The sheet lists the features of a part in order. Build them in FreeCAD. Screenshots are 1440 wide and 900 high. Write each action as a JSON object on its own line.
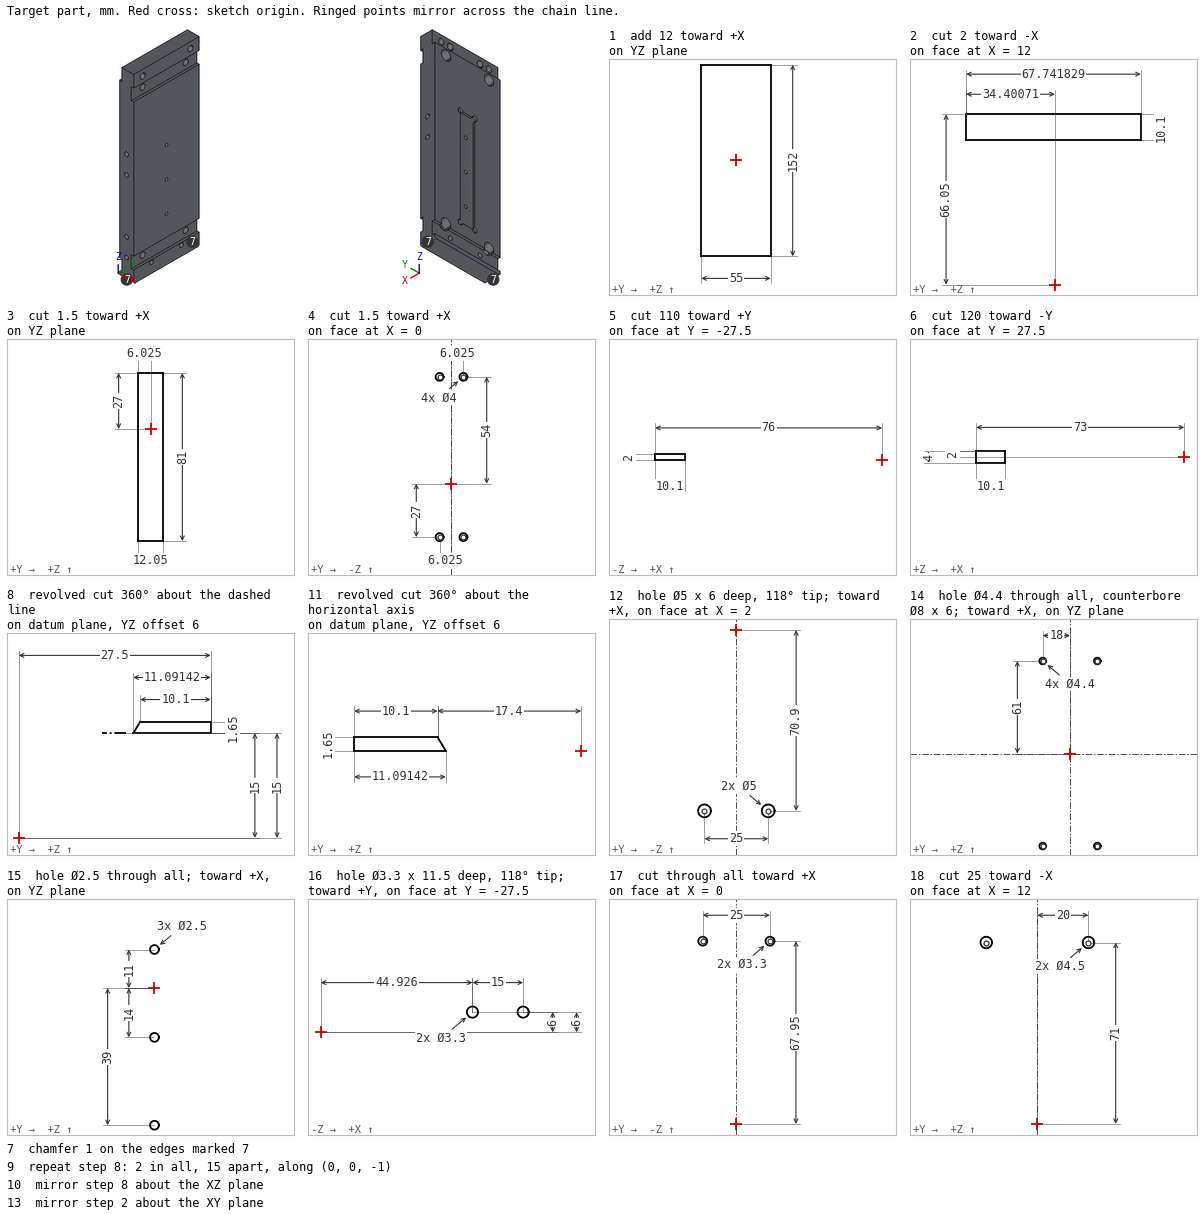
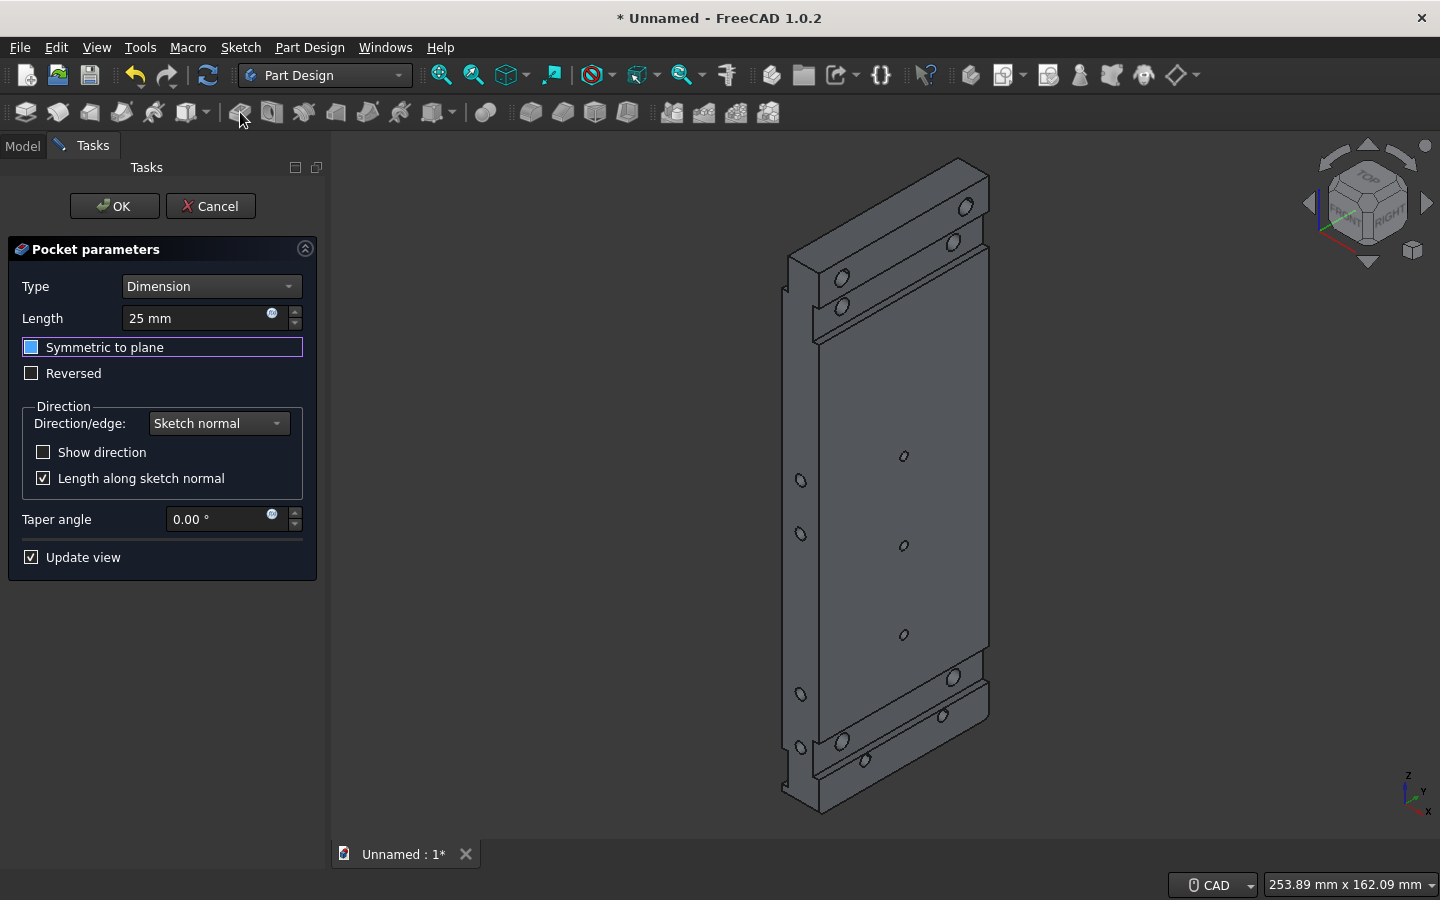
{"action": "left_click", "coordinate": [115, 206]}